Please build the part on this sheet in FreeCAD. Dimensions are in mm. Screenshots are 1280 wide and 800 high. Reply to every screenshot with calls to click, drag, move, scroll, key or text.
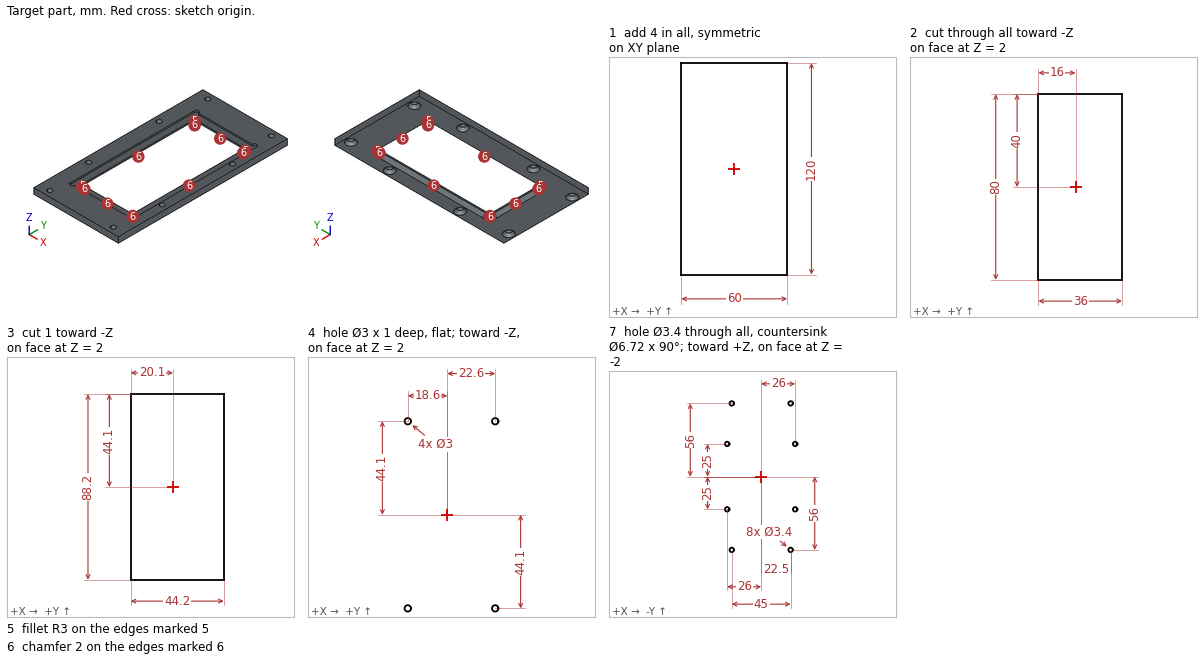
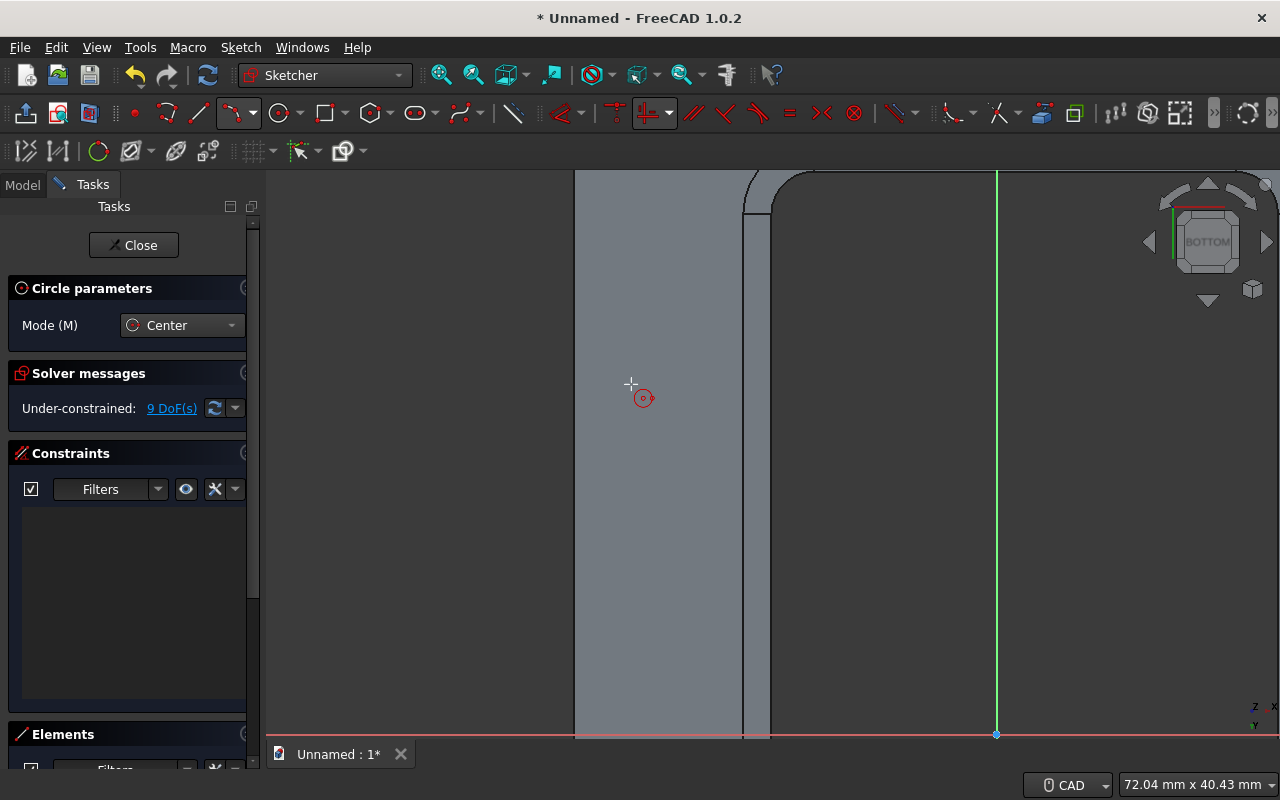
scroll(631, 384, down, 8)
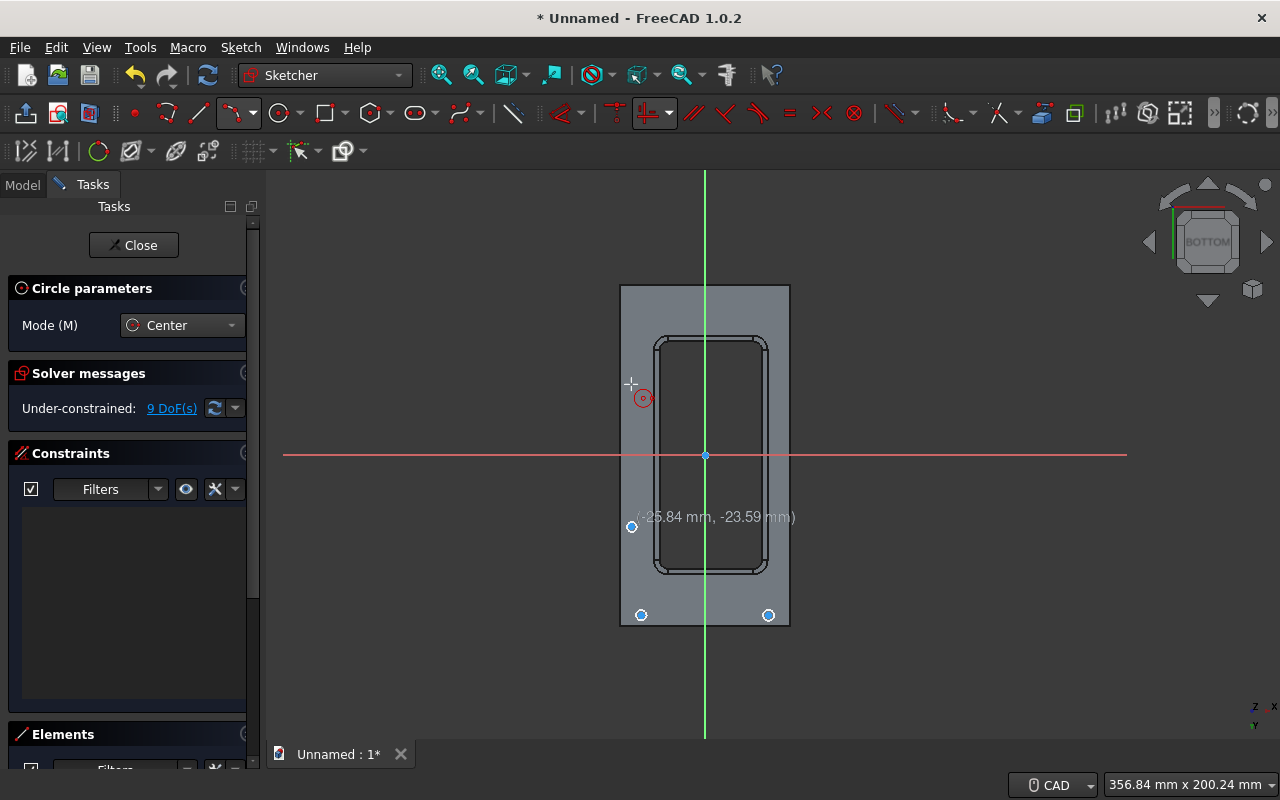
click(631, 384)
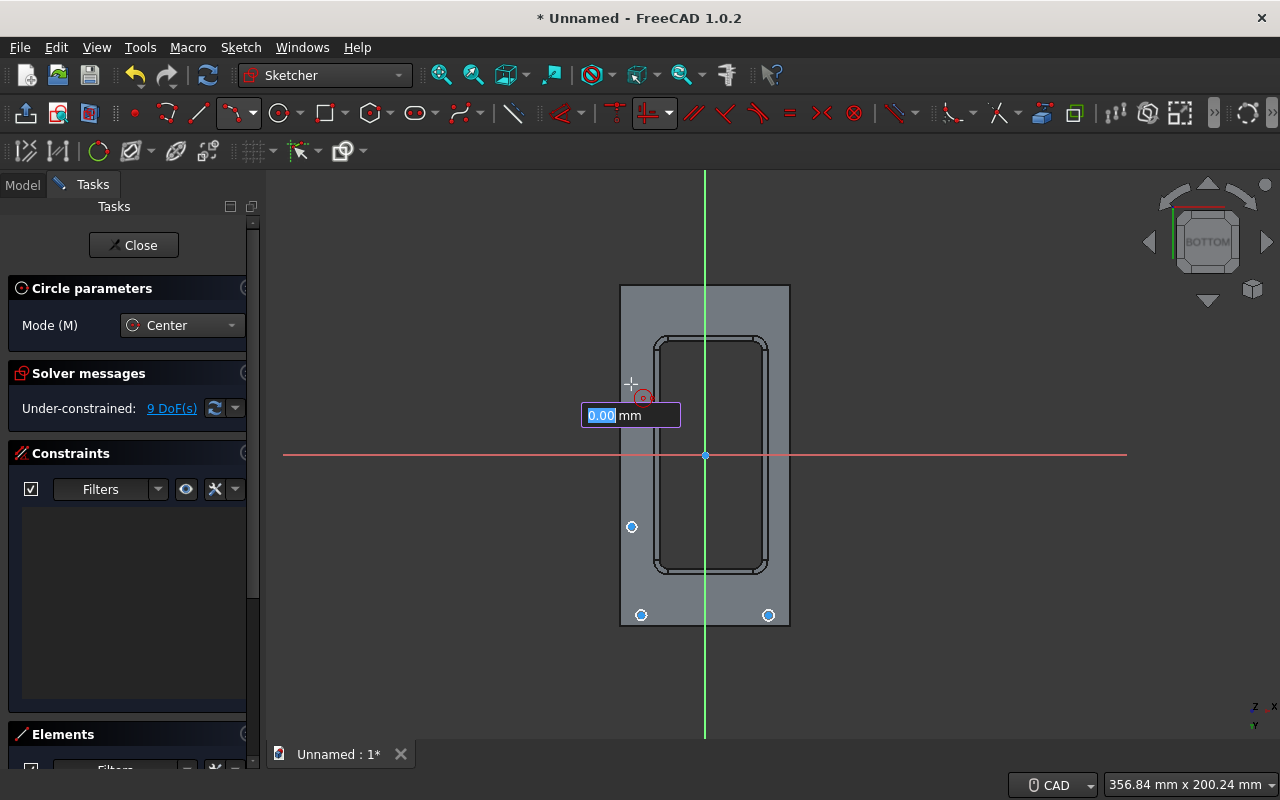
scroll(635, 381, up, 6)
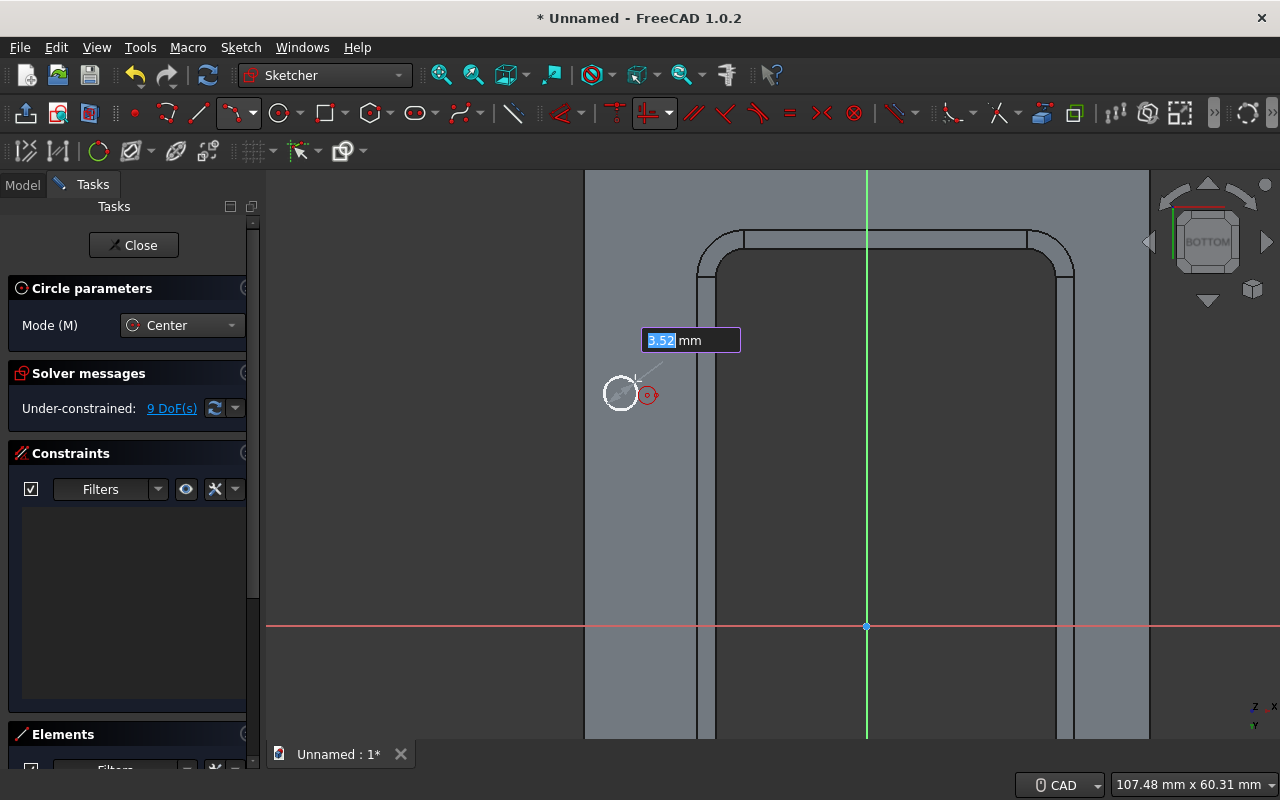
click(633, 379)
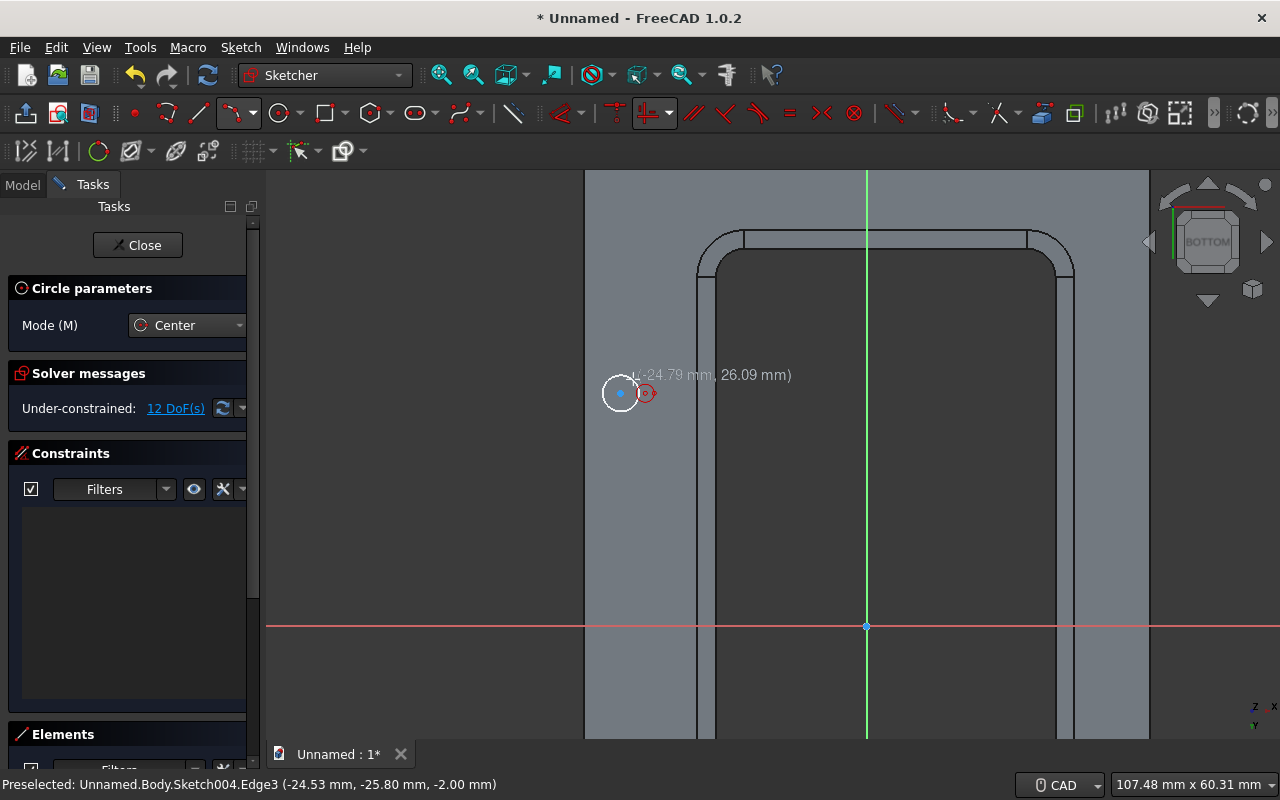
scroll(635, 381, down, 6)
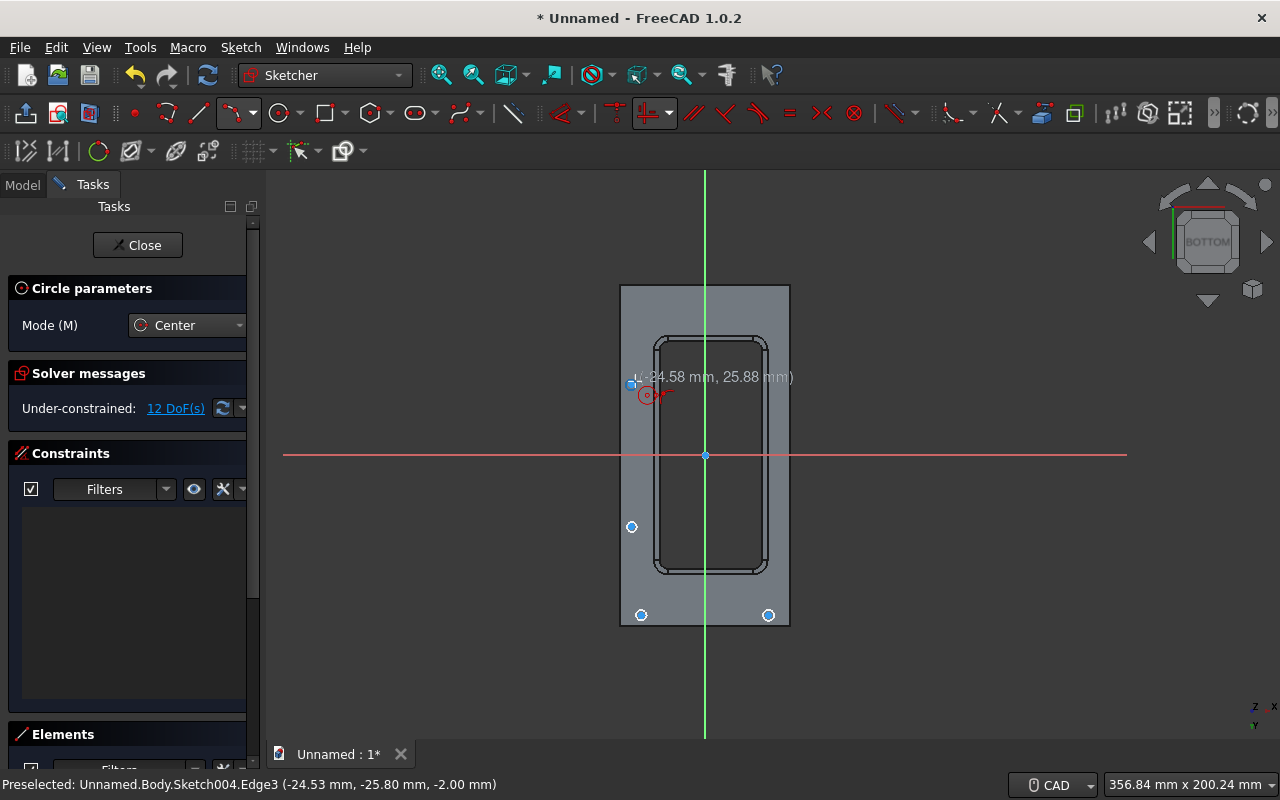
scroll(641, 296, up, 8)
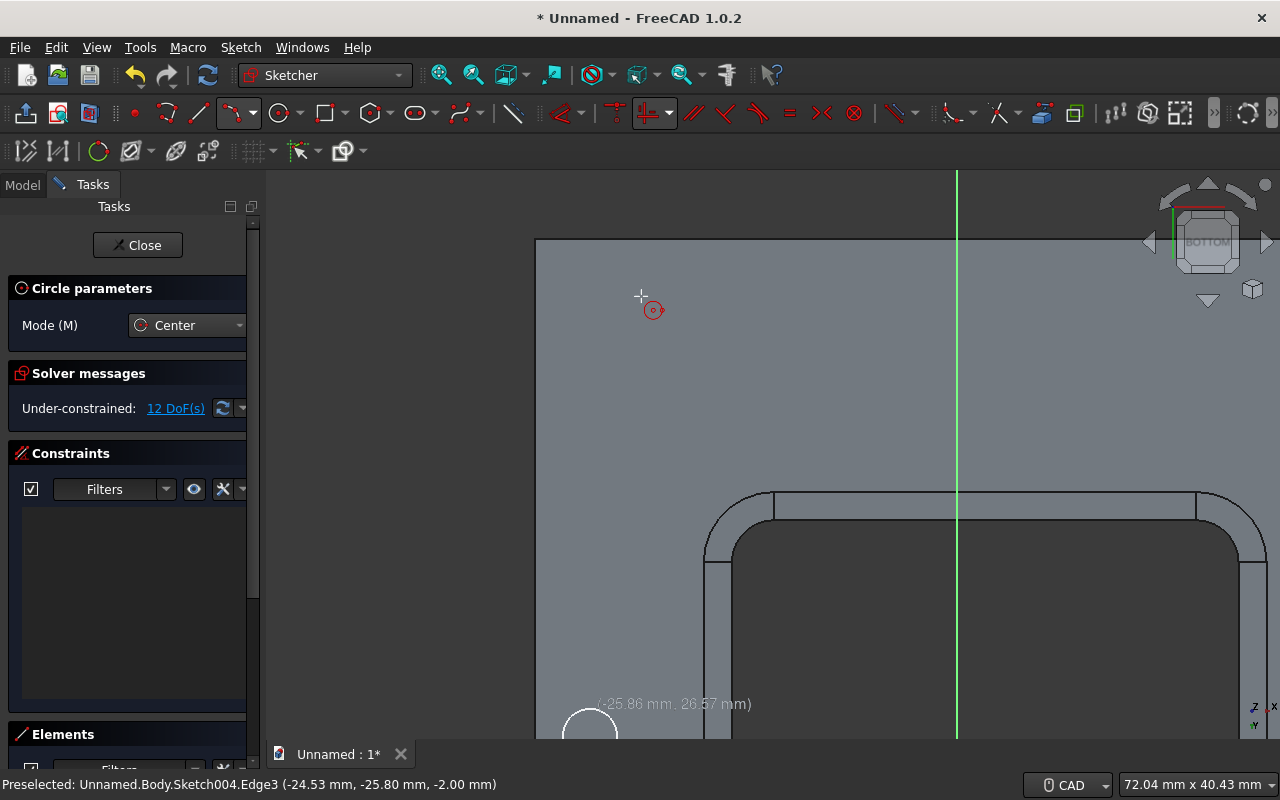
scroll(641, 295, down, 8)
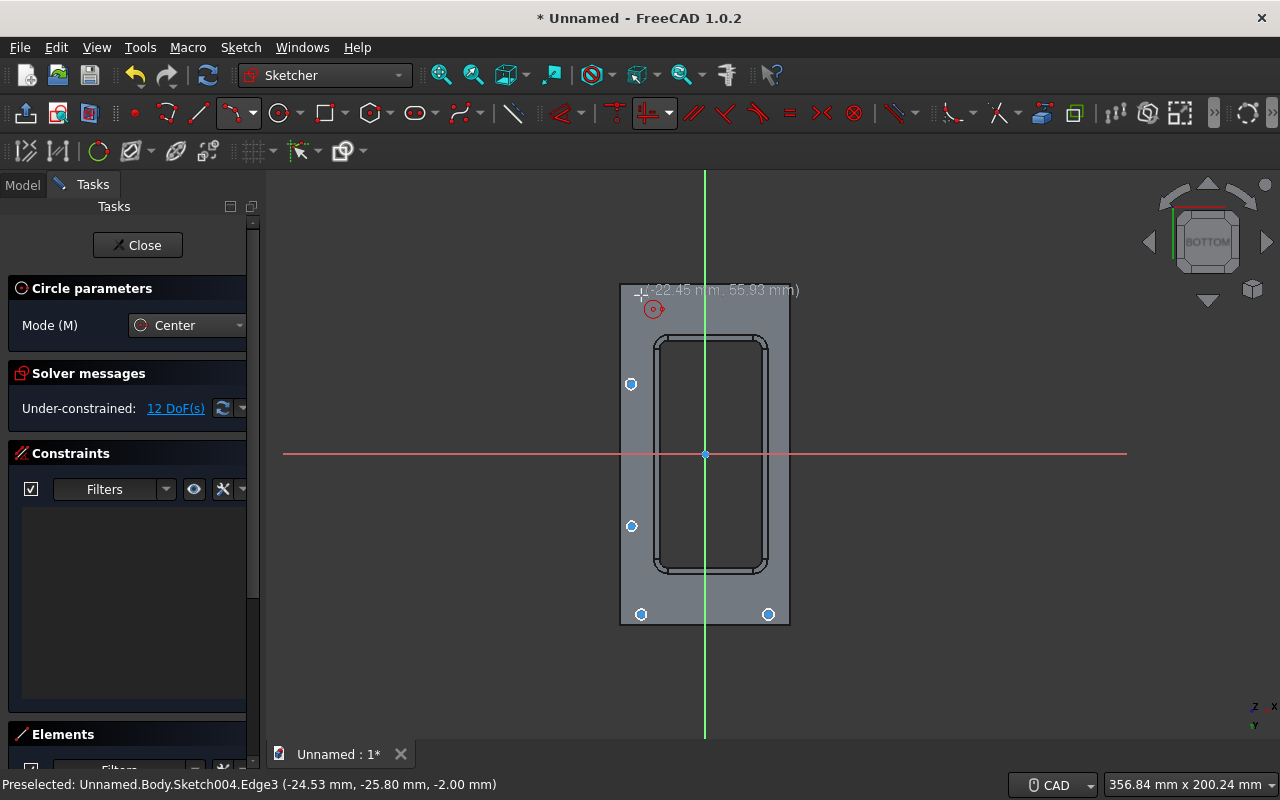
click(641, 295)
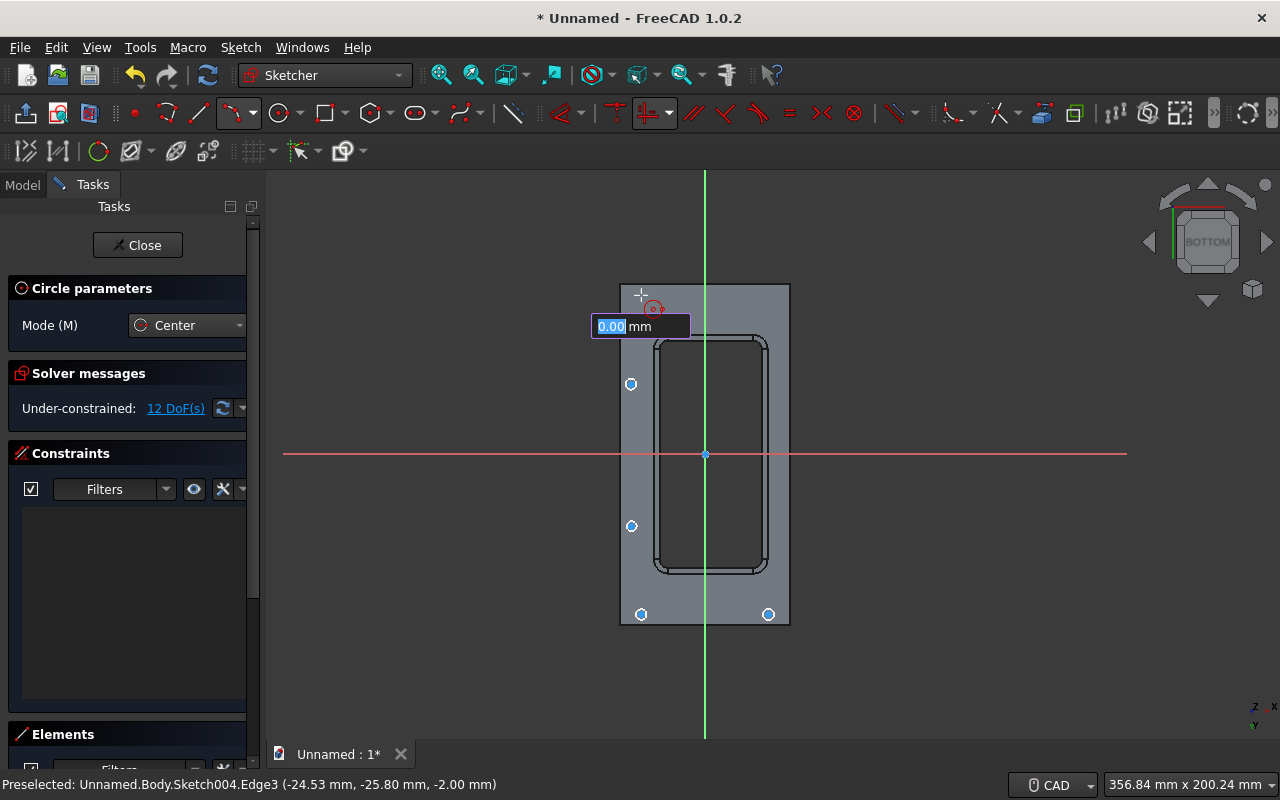
scroll(645, 292, up, 6)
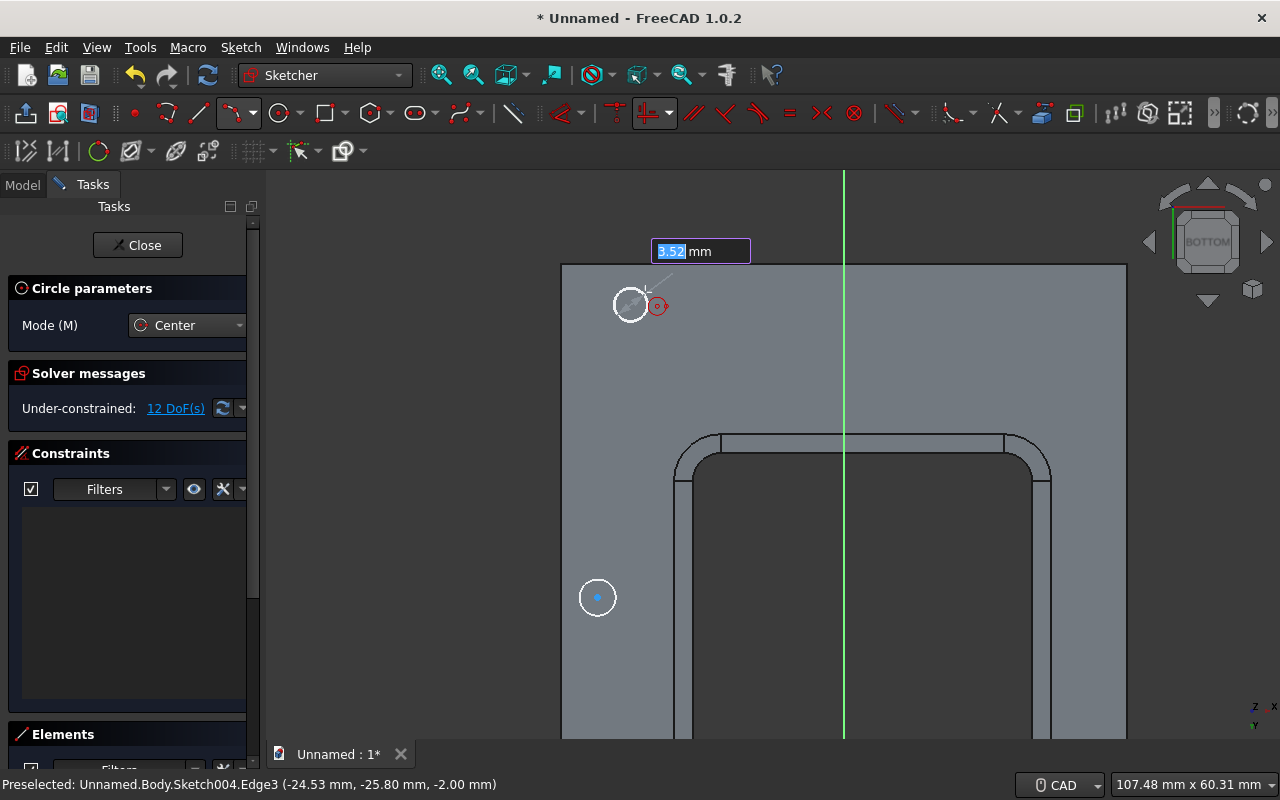
click(643, 291)